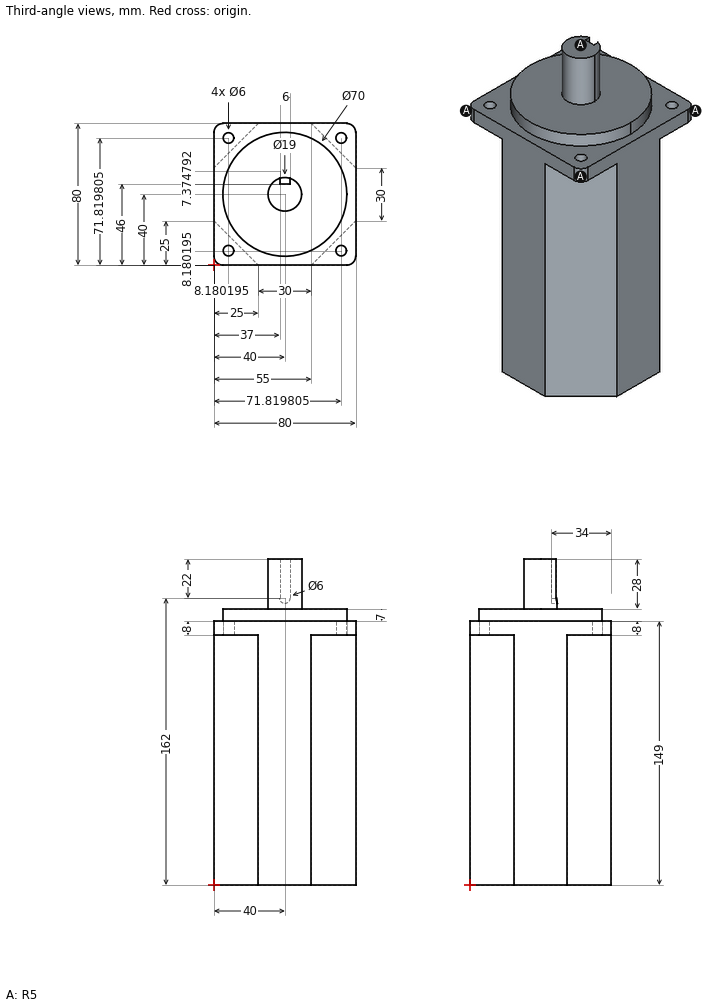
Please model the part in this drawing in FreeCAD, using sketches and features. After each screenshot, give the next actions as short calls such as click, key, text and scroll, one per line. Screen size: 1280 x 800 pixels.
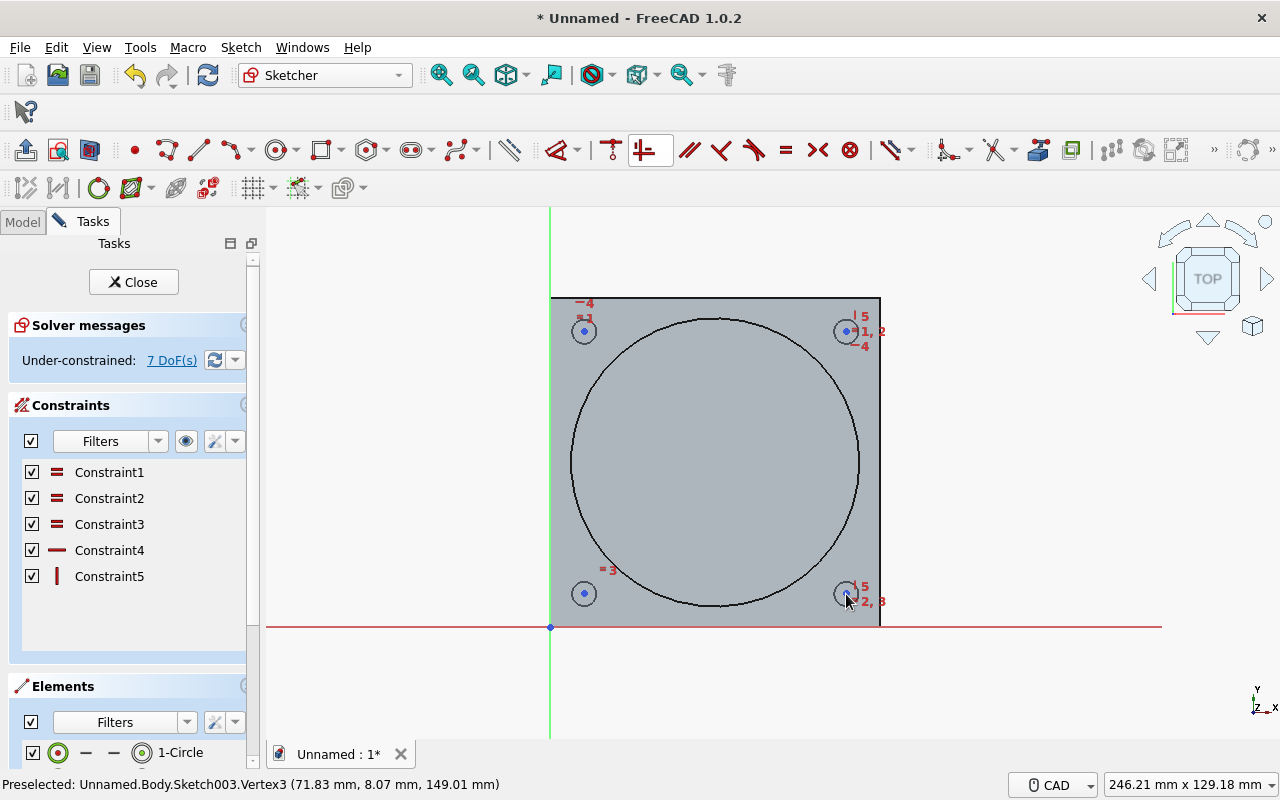
click(584, 332)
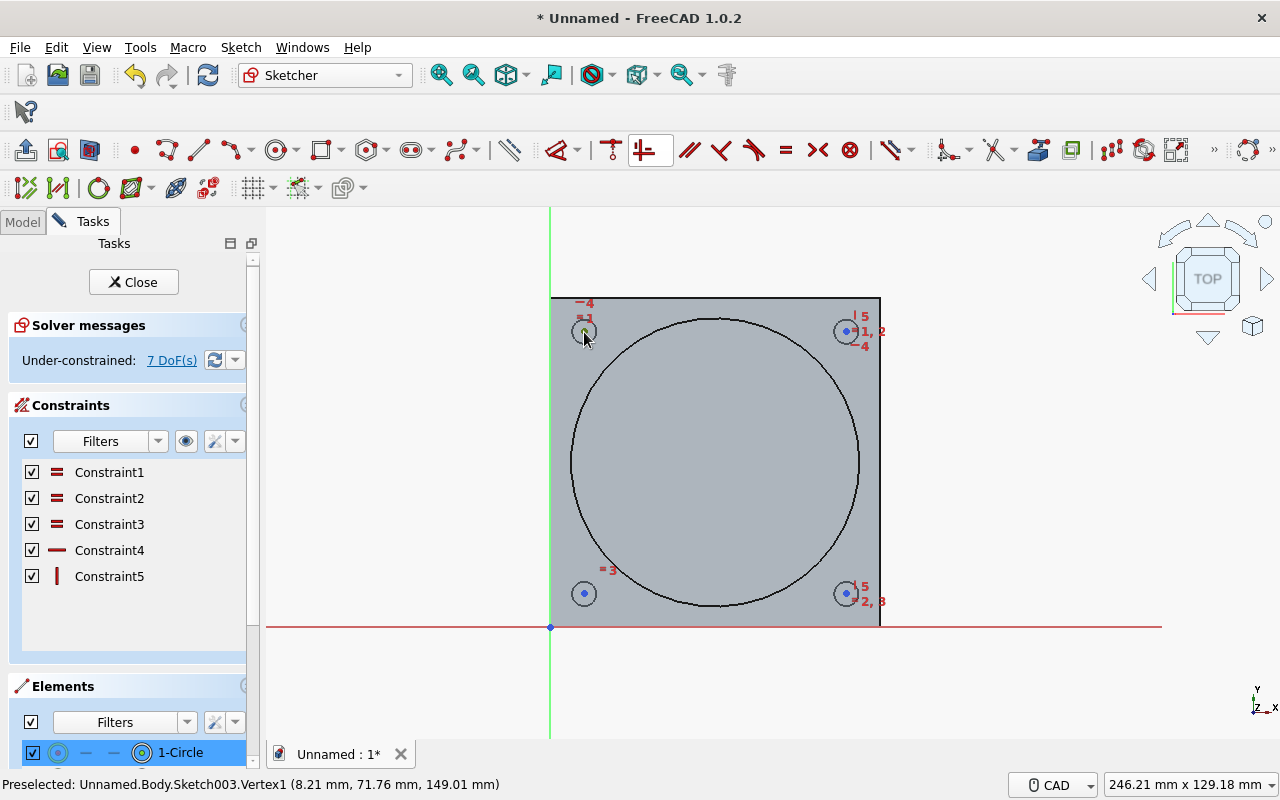
click(584, 594)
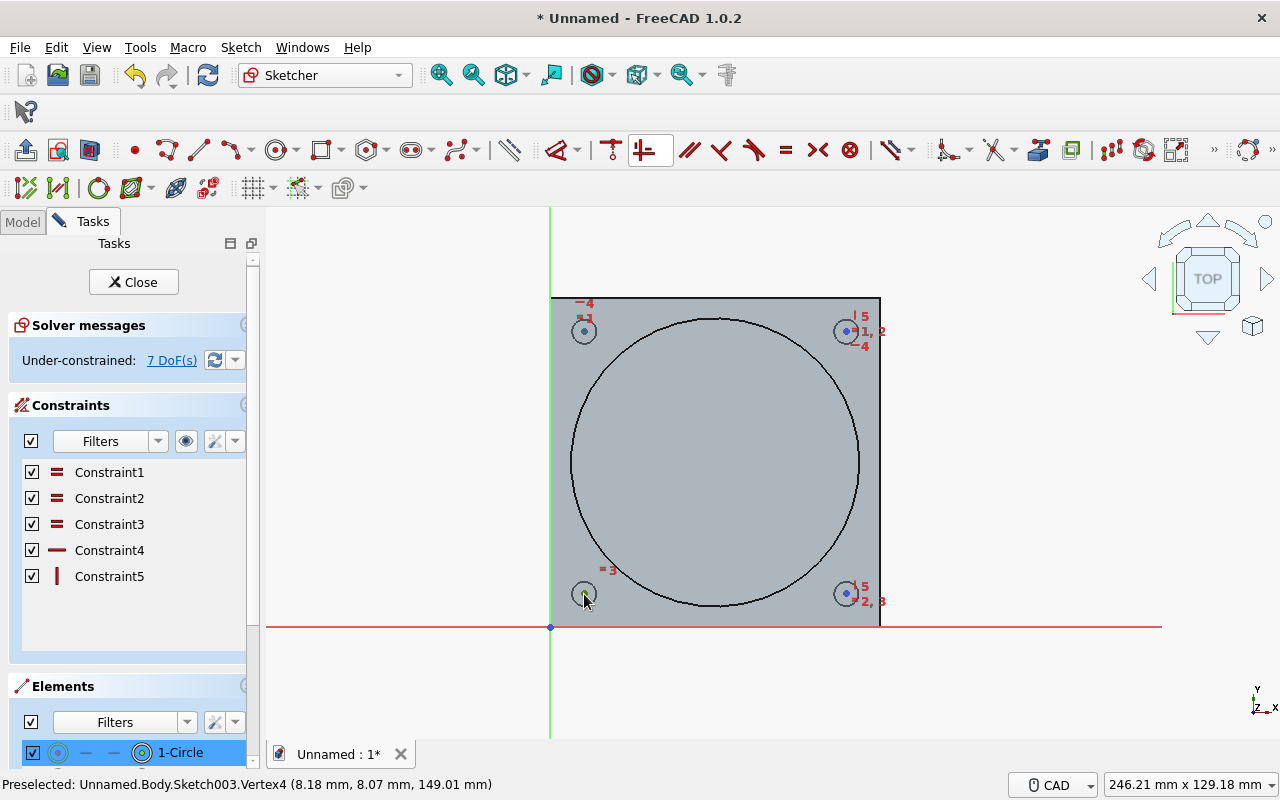
key(v)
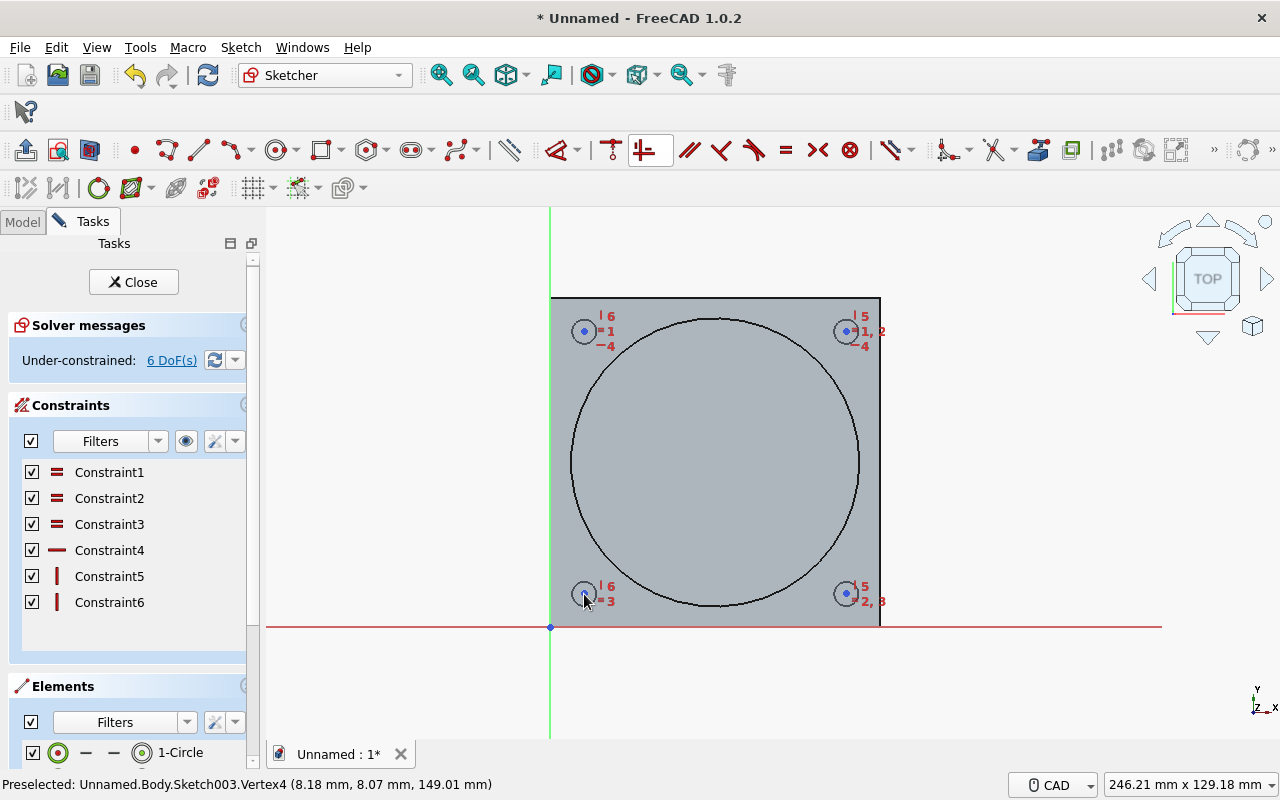
click(846, 594)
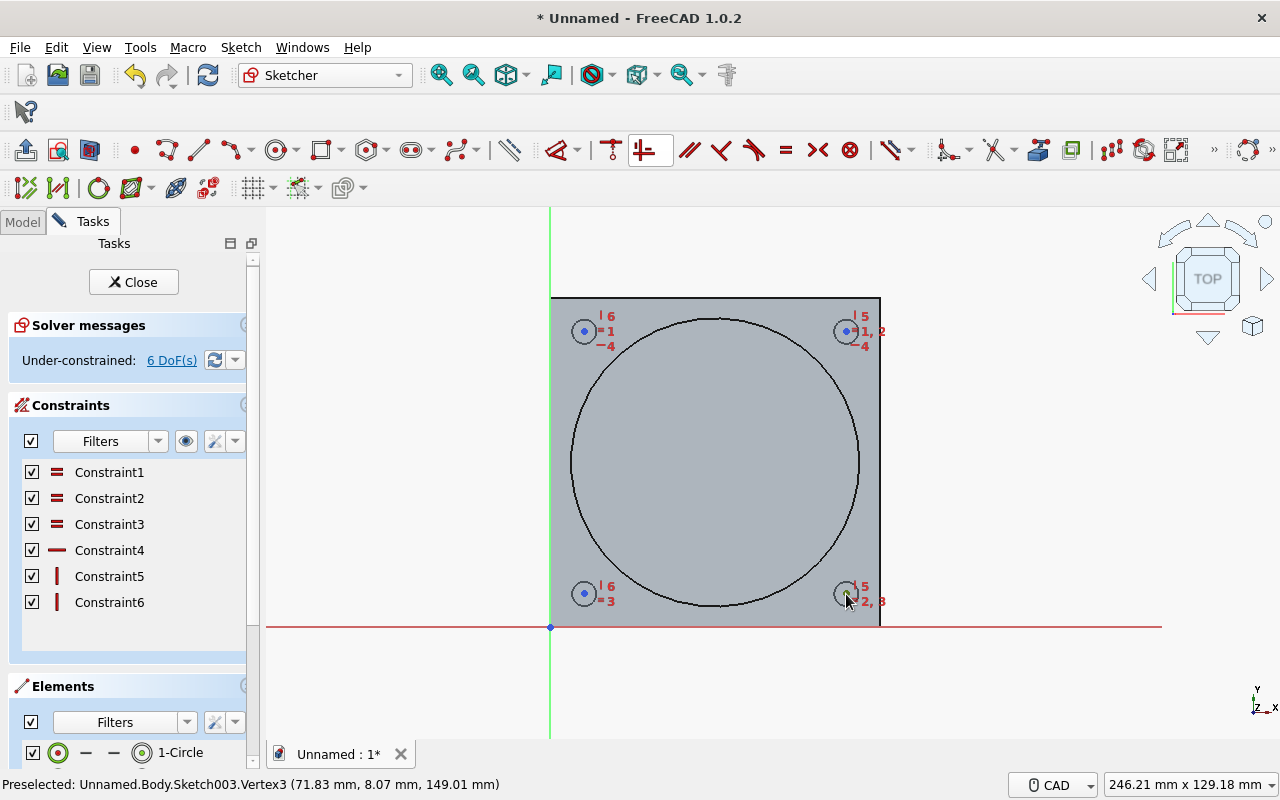
click(584, 594)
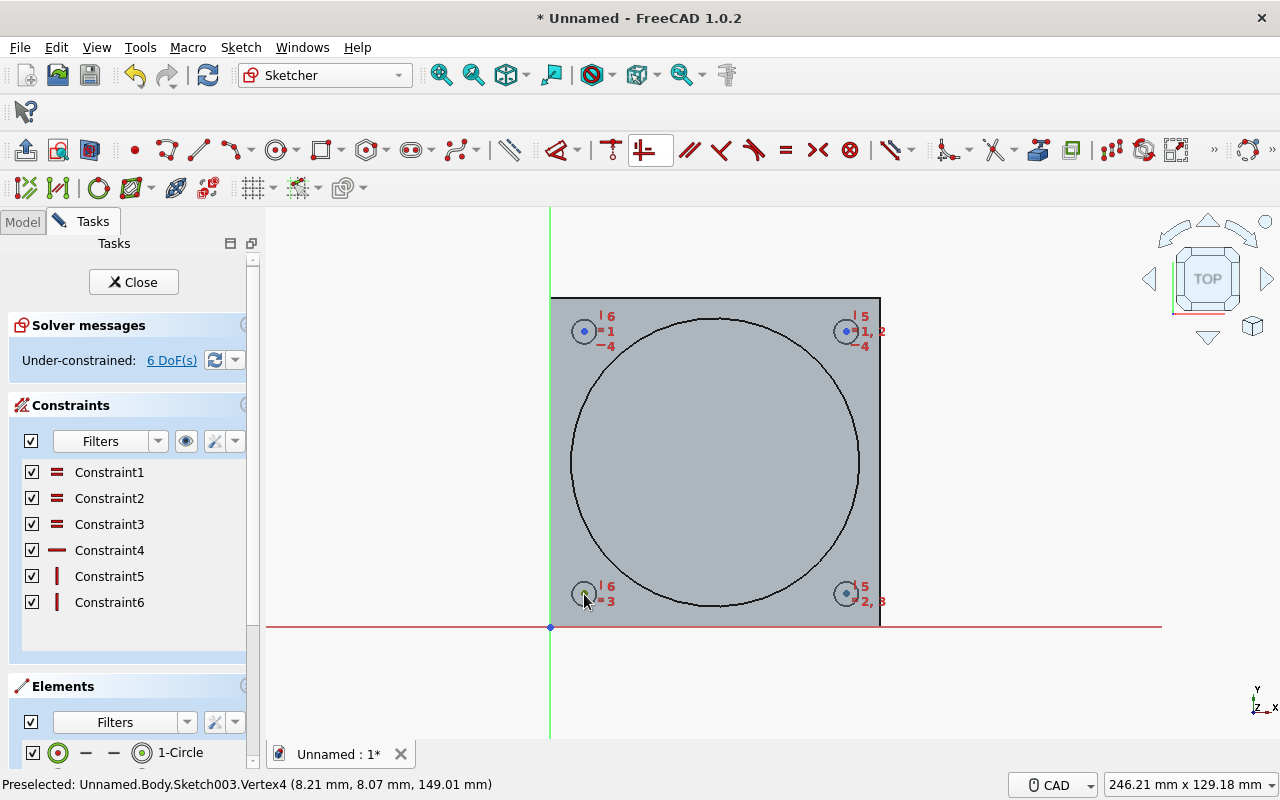
key(h)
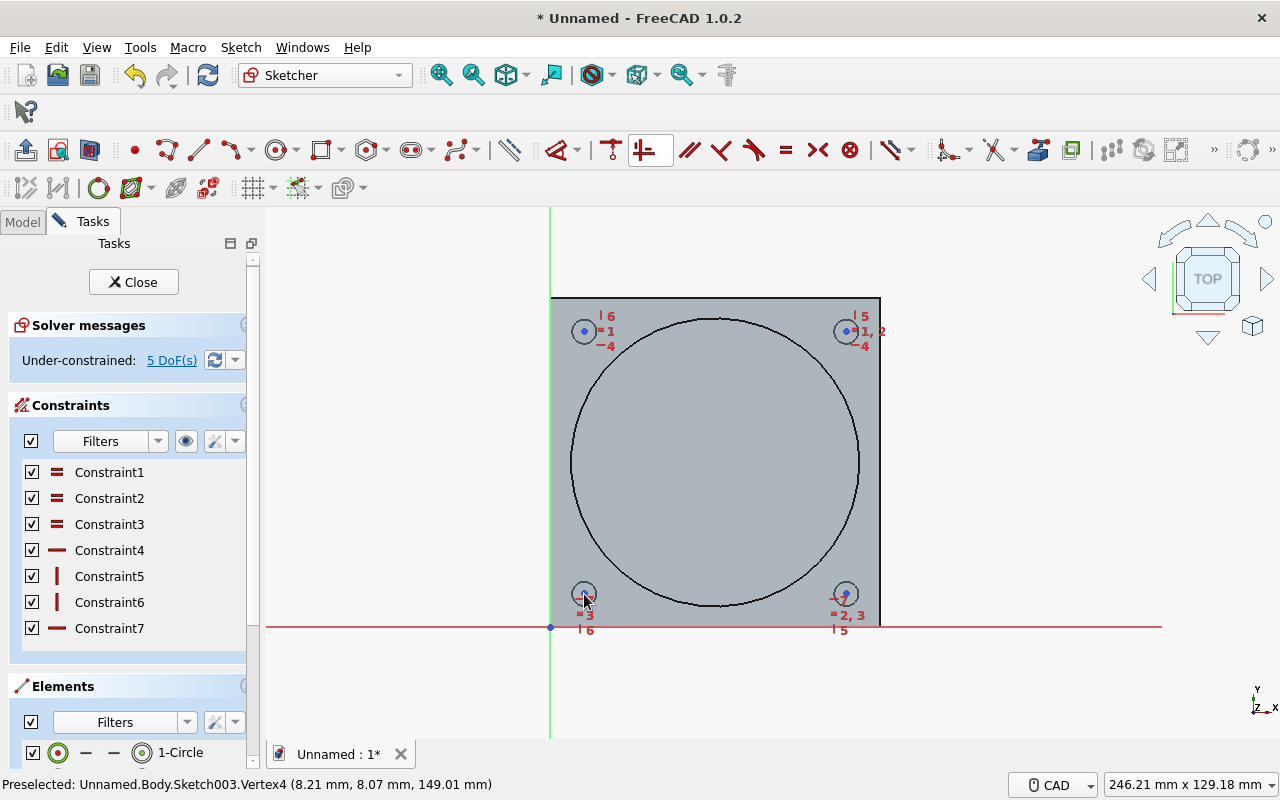
click(556, 150)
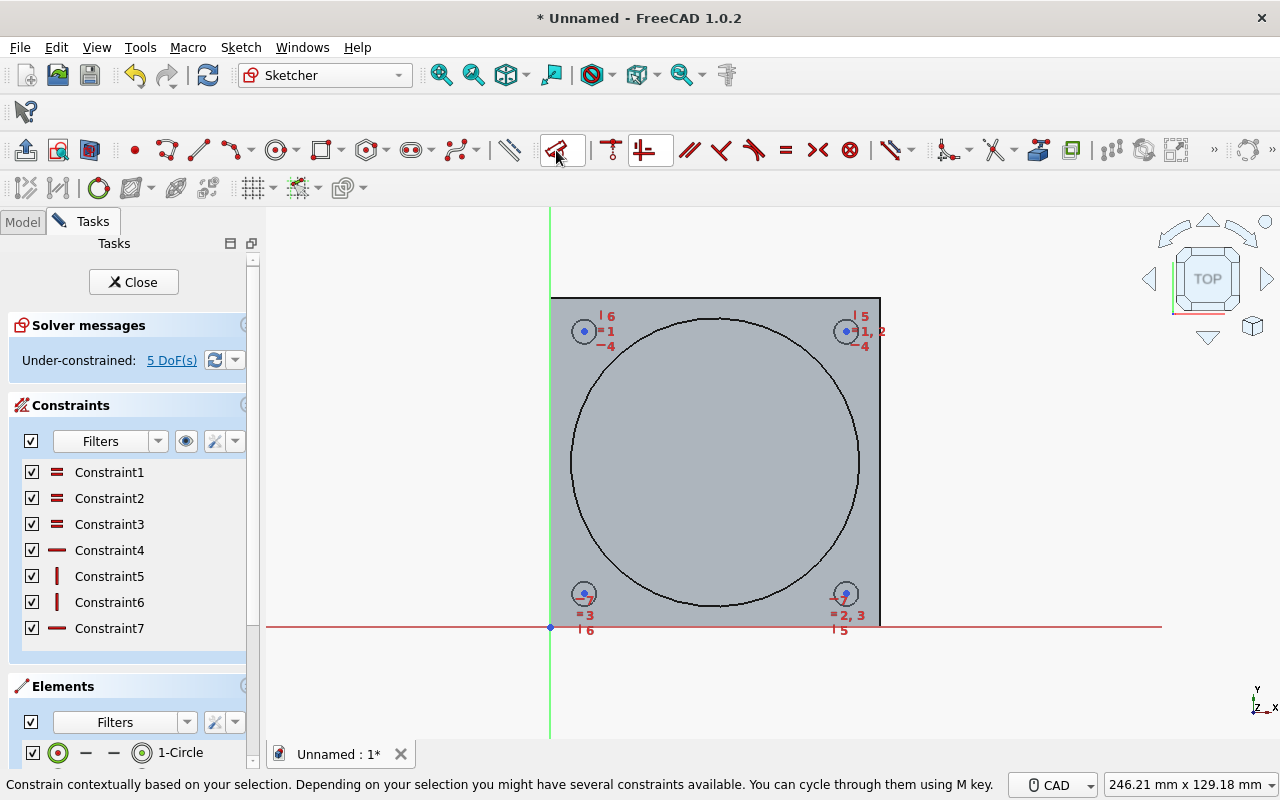
scroll(593, 323, up, 3)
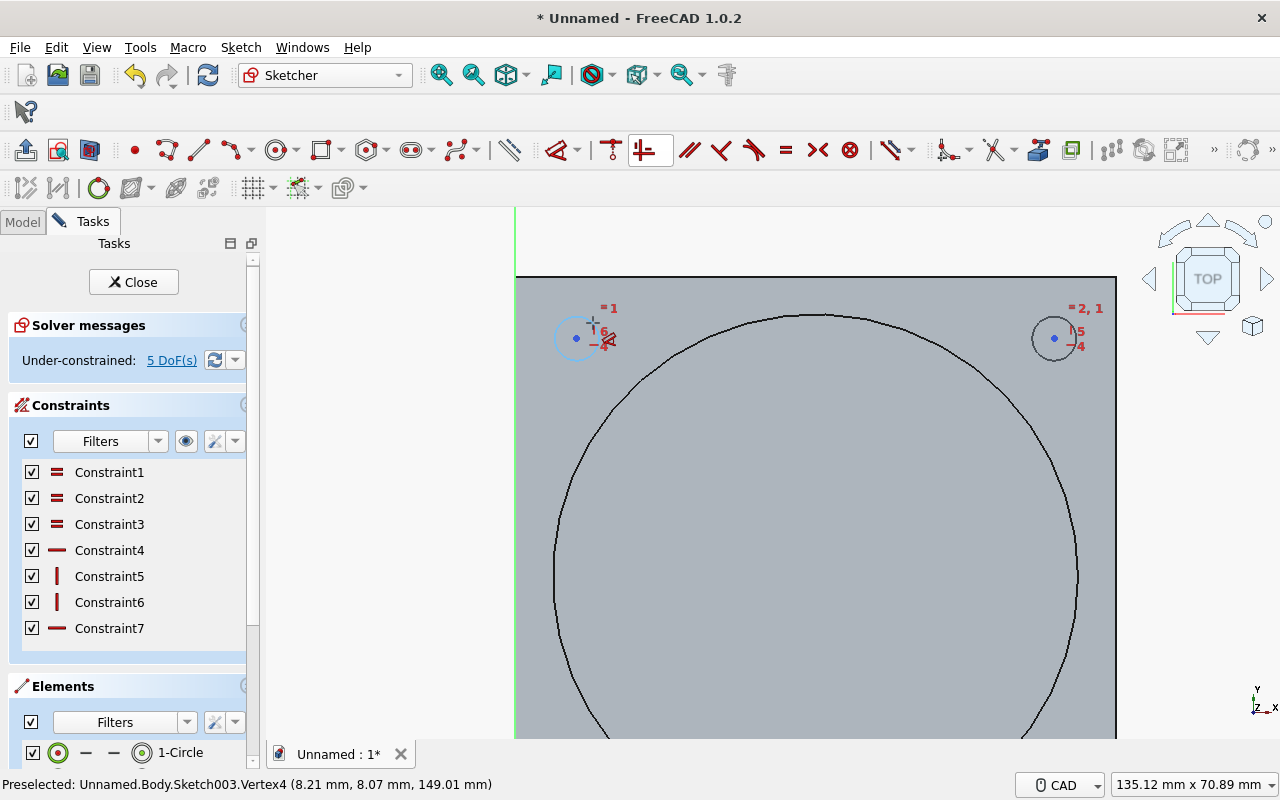
click(592, 323)
click(614, 300)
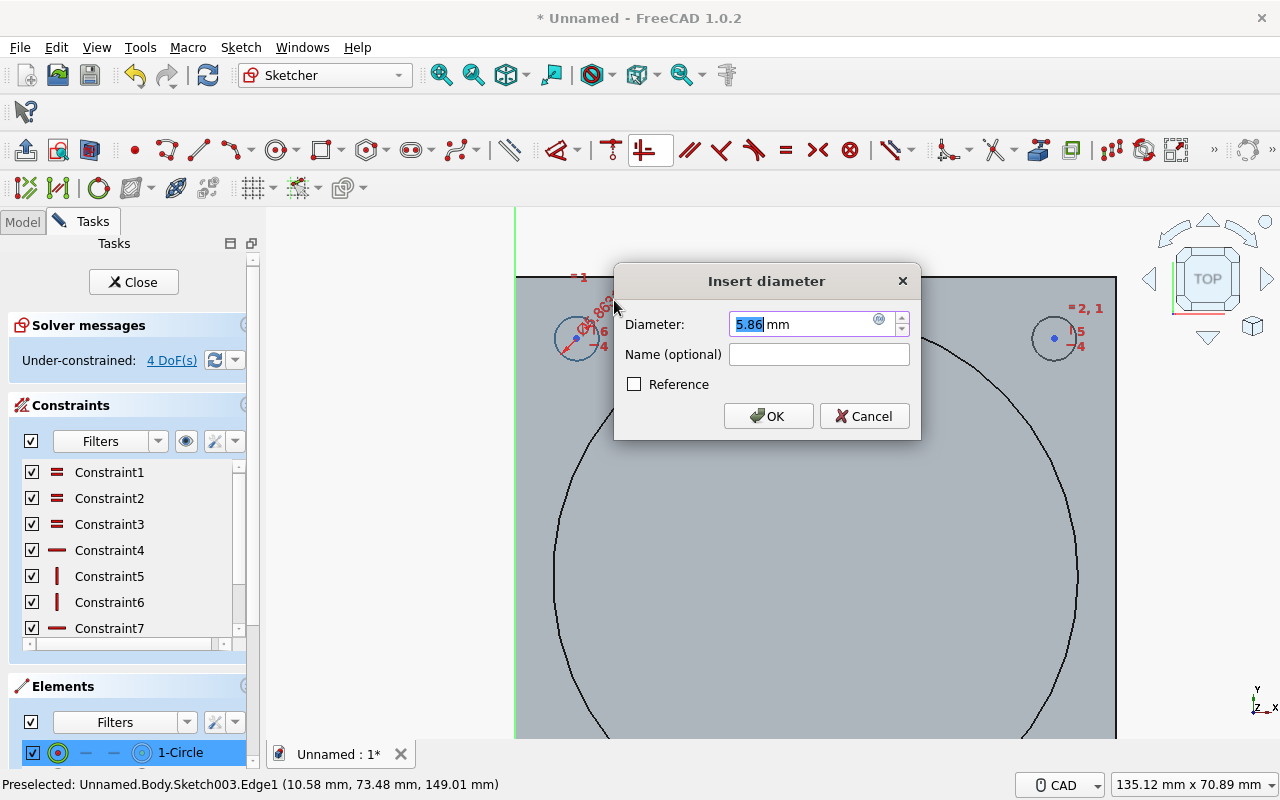
text(6)
key(Return)